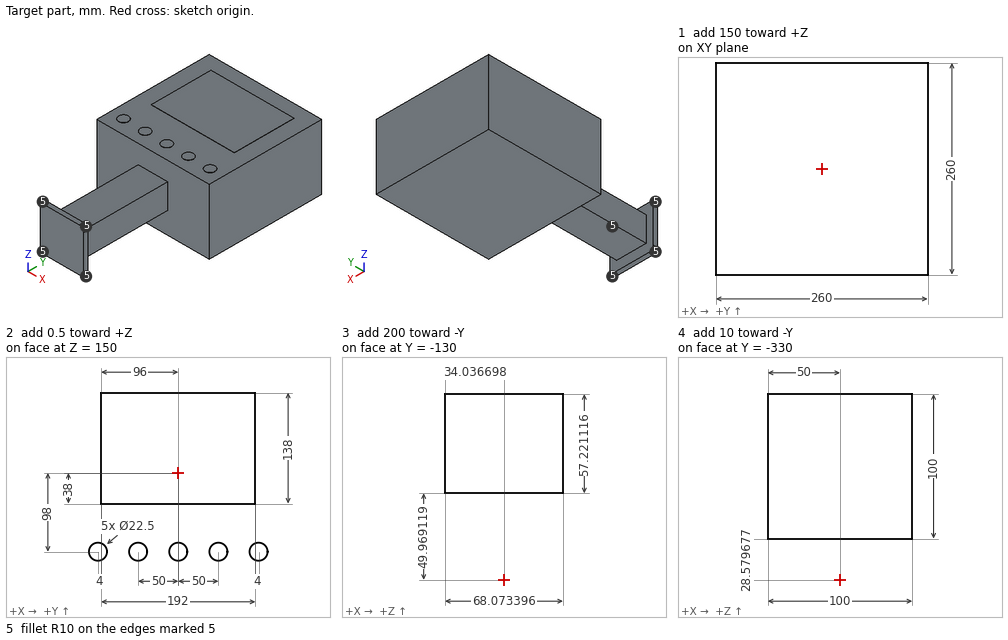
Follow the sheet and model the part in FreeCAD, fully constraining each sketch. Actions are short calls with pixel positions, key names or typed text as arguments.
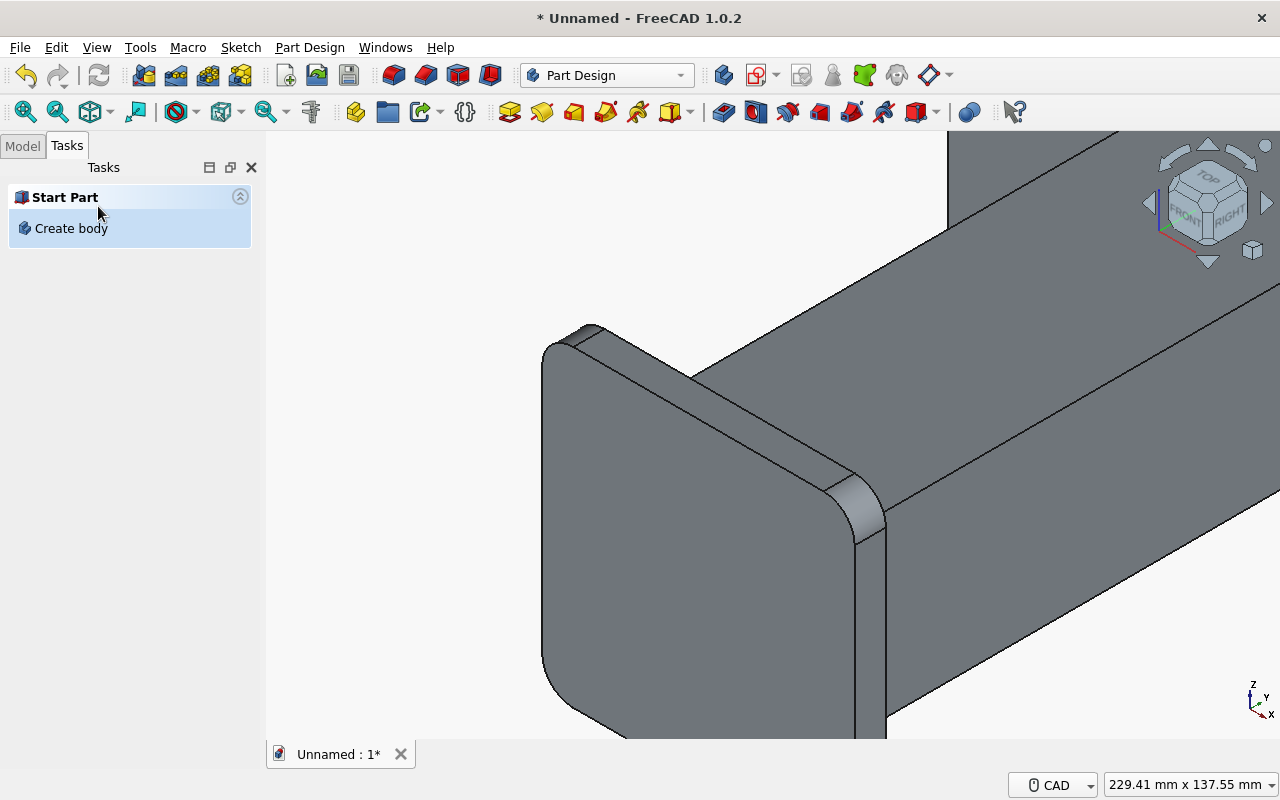
key(v)
key(f)